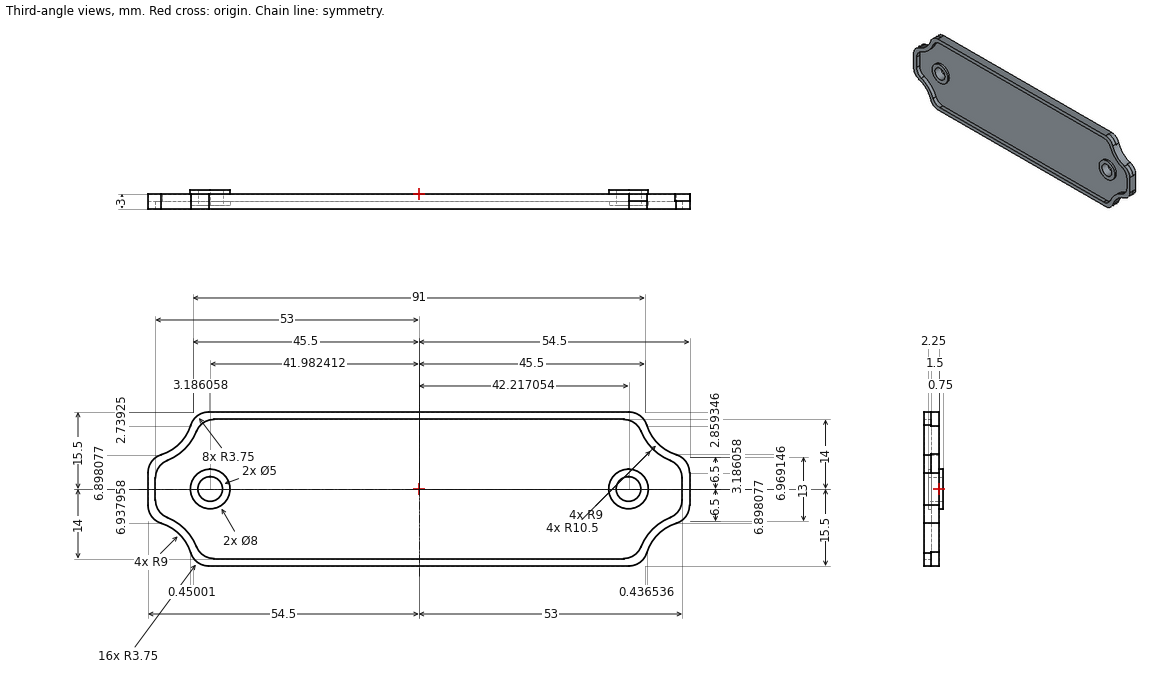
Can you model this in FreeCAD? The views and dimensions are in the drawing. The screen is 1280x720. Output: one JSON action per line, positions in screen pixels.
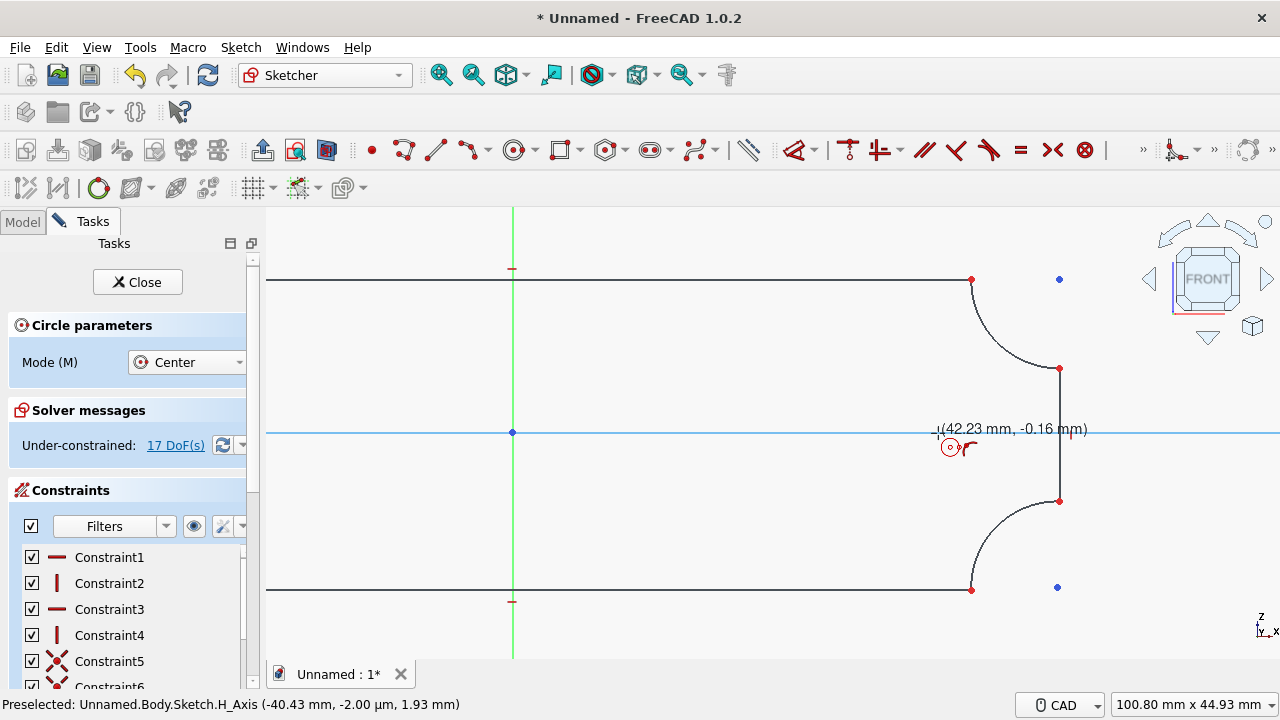
{"action": "left_click", "coordinate": [937, 433]}
{"action": "mouse_move", "coordinate": [955, 415]}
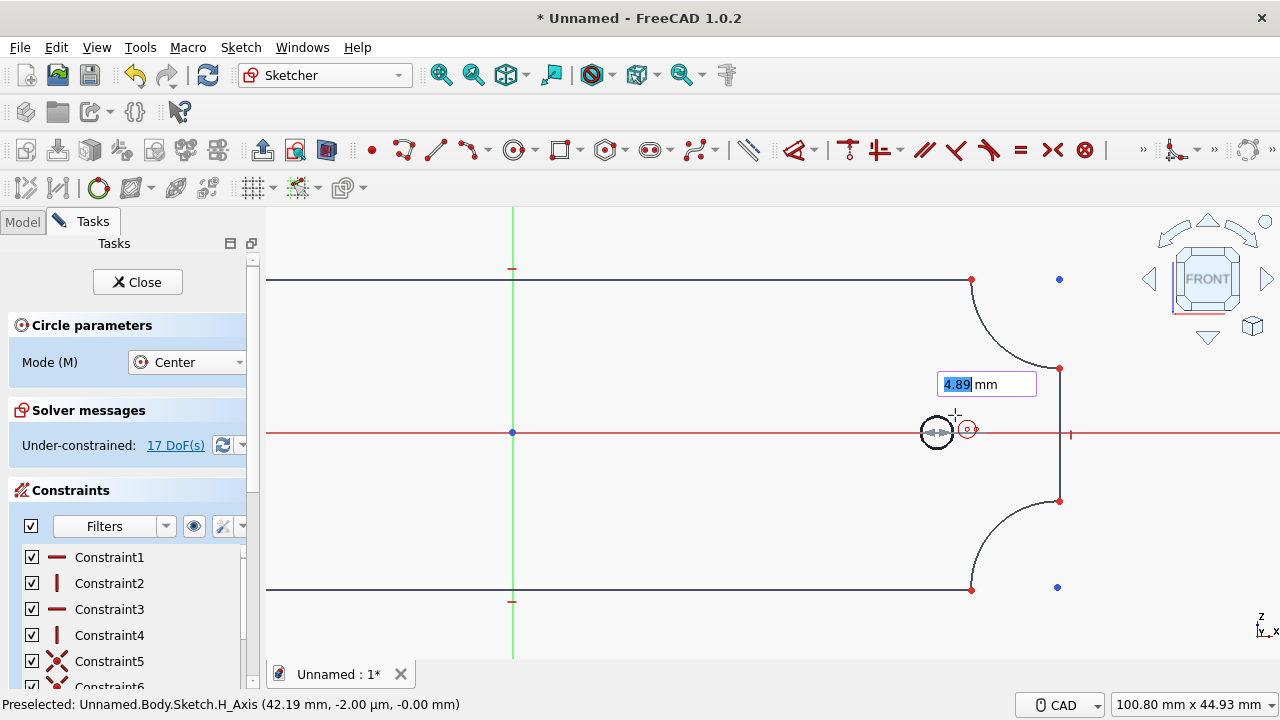
{"action": "type", "text": "5"}
{"action": "key", "text": "Return"}
{"action": "key", "text": "Escape"}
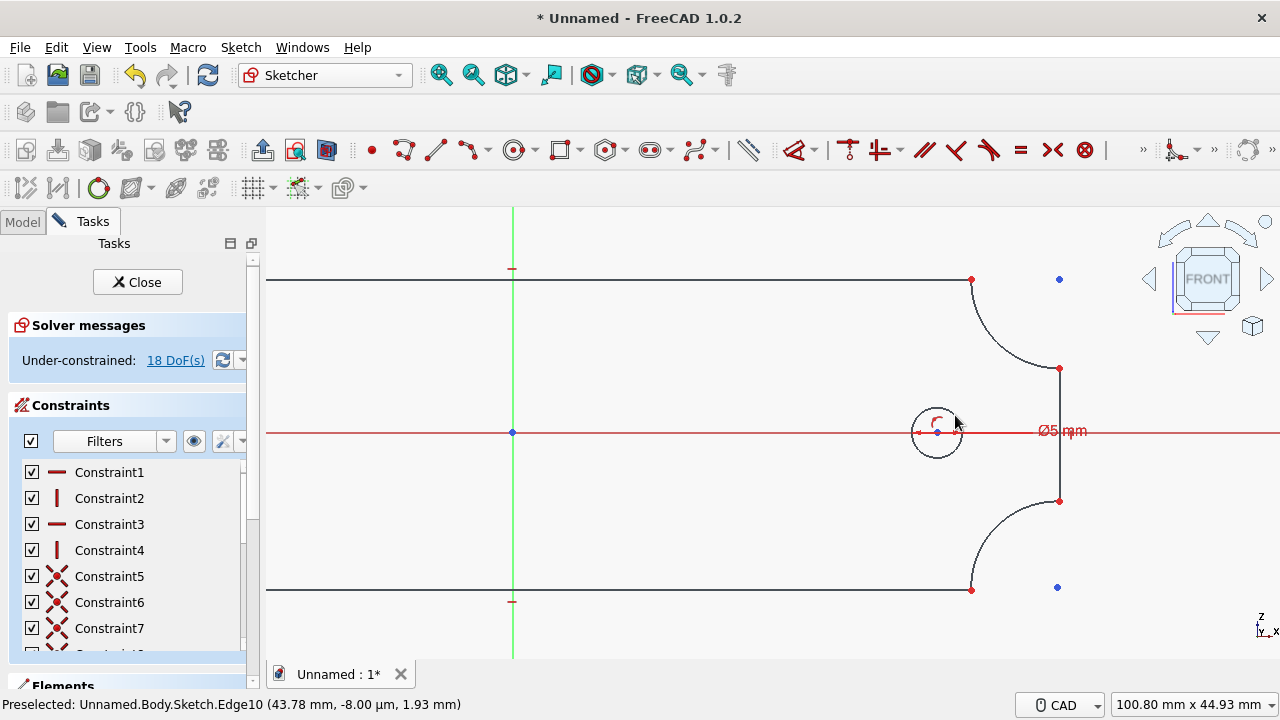
{"action": "left_click", "coordinate": [981, 320]}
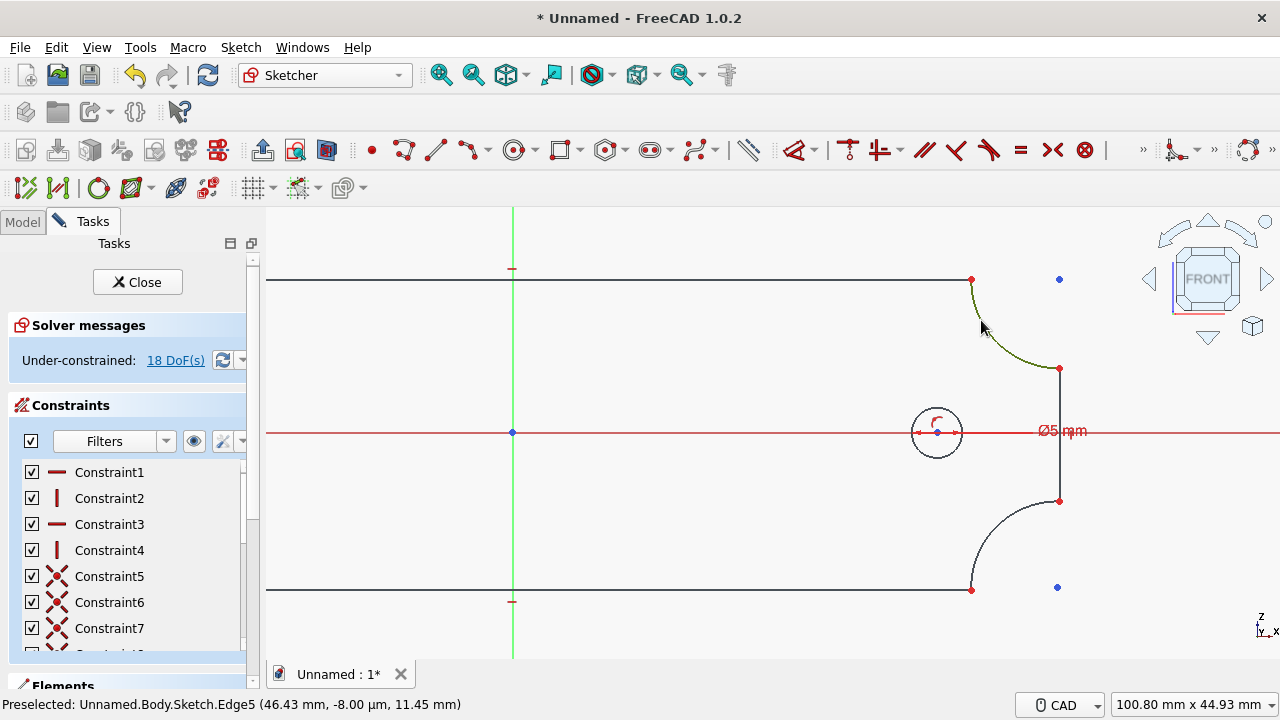
{"action": "left_click", "coordinate": [1019, 510]}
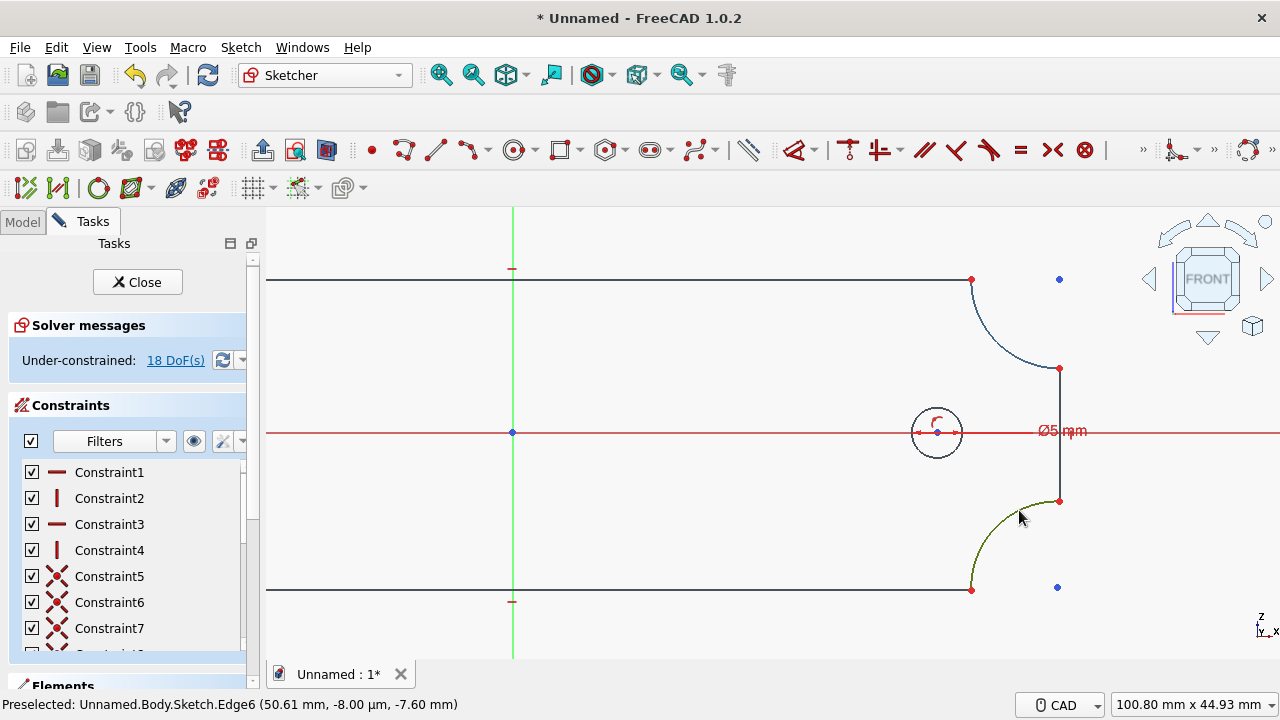
{"action": "scroll", "coordinate": [938, 433], "scroll_direction": "down", "scroll_amount": 3}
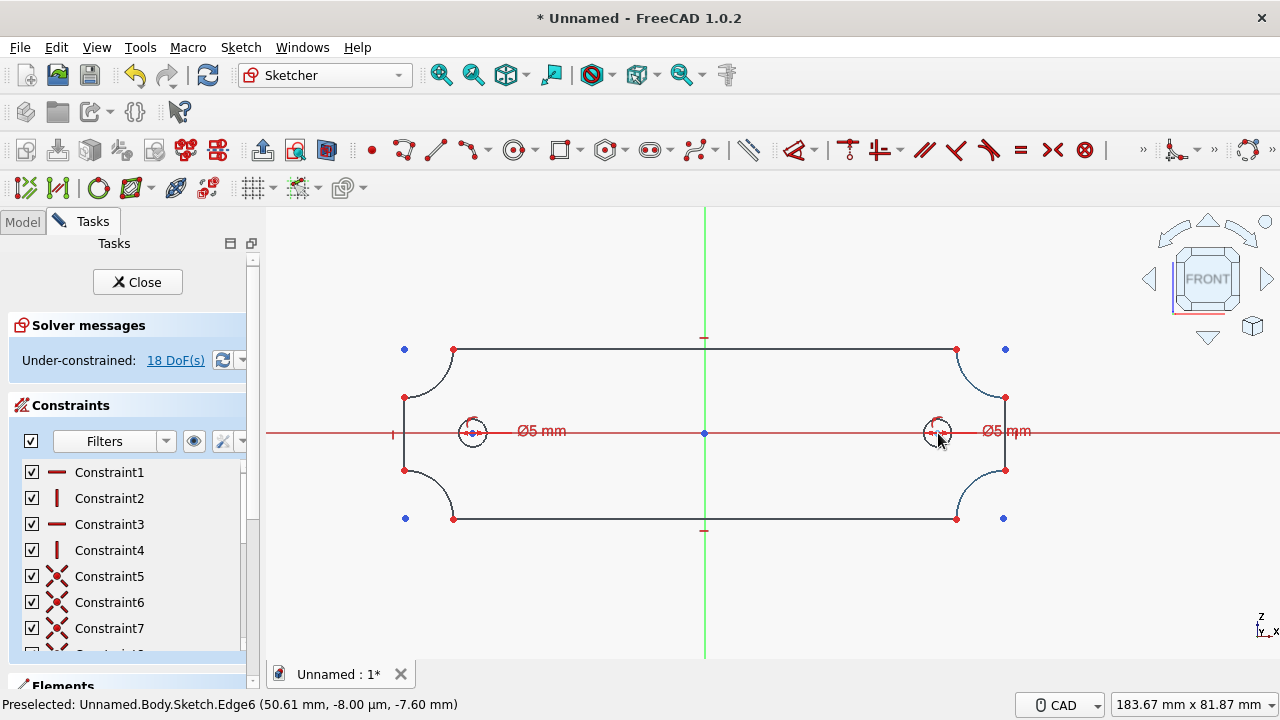
{"action": "left_click", "coordinate": [448, 497]}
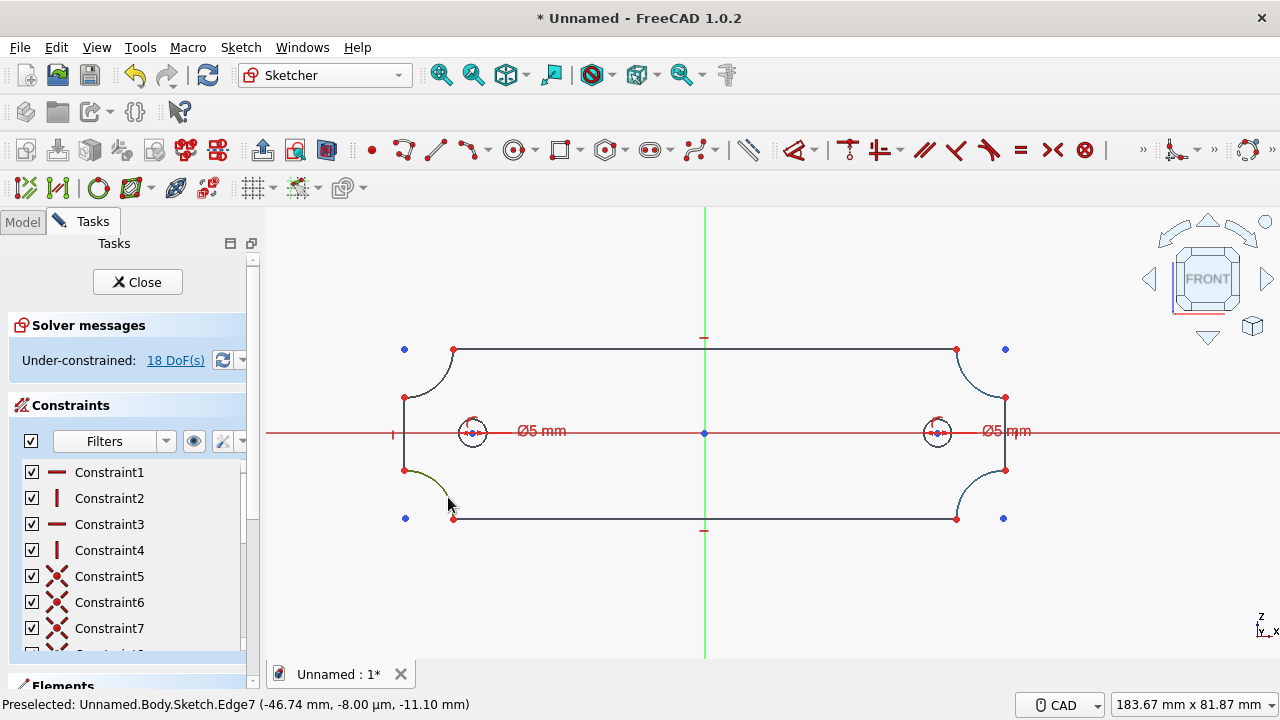
{"action": "left_click", "coordinate": [427, 393]}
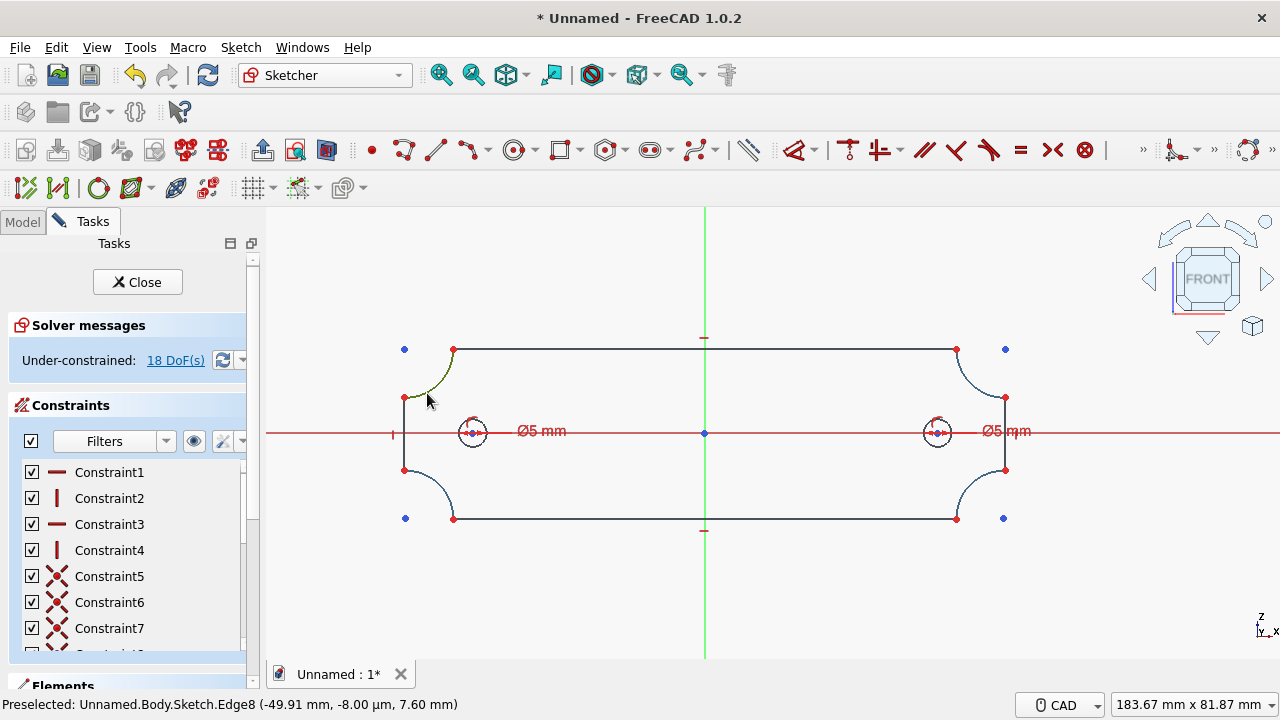
{"action": "left_click", "coordinate": [1022, 150]}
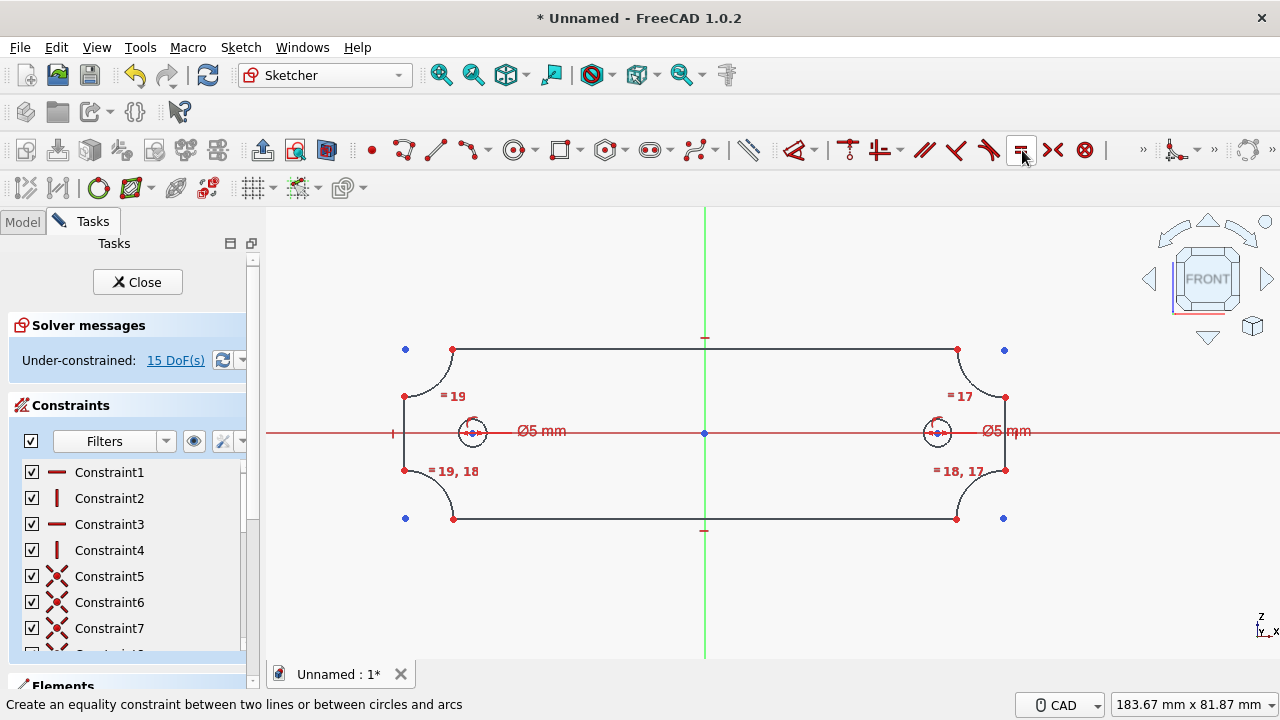
{"action": "left_click", "coordinate": [1005, 350]}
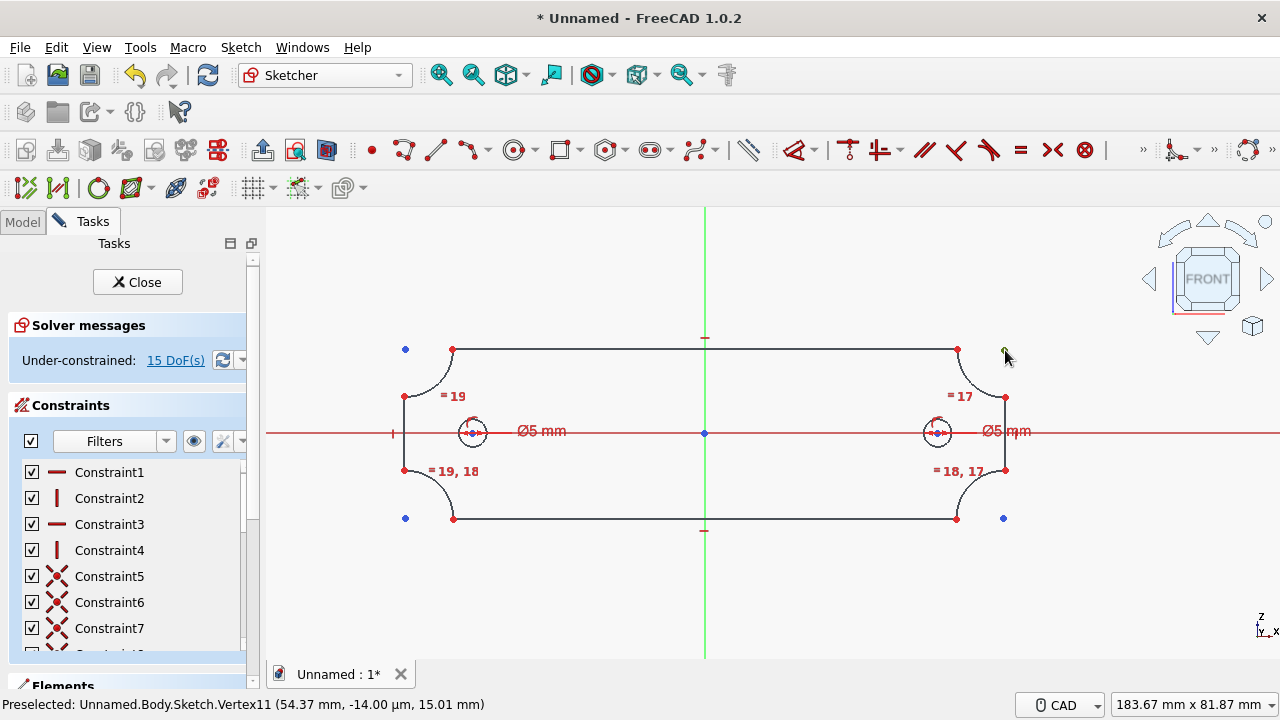
{"action": "left_click", "coordinate": [1004, 518]}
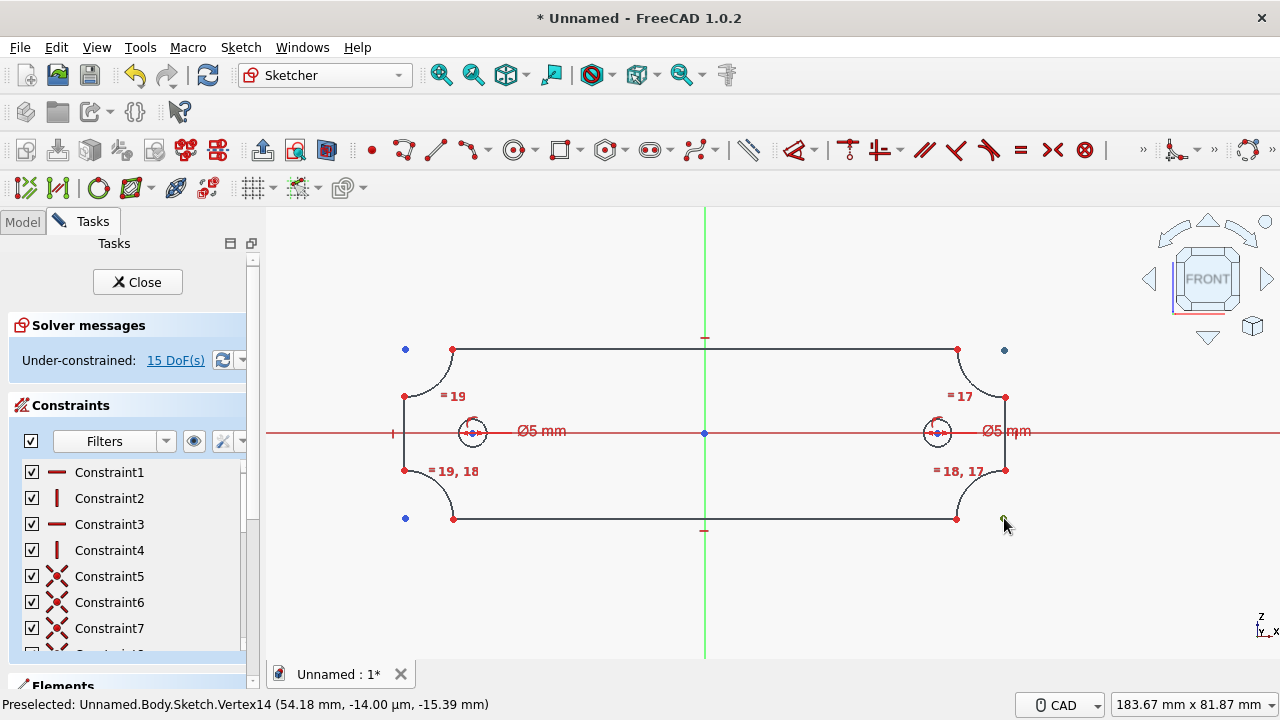
{"action": "left_click", "coordinate": [353, 433]}